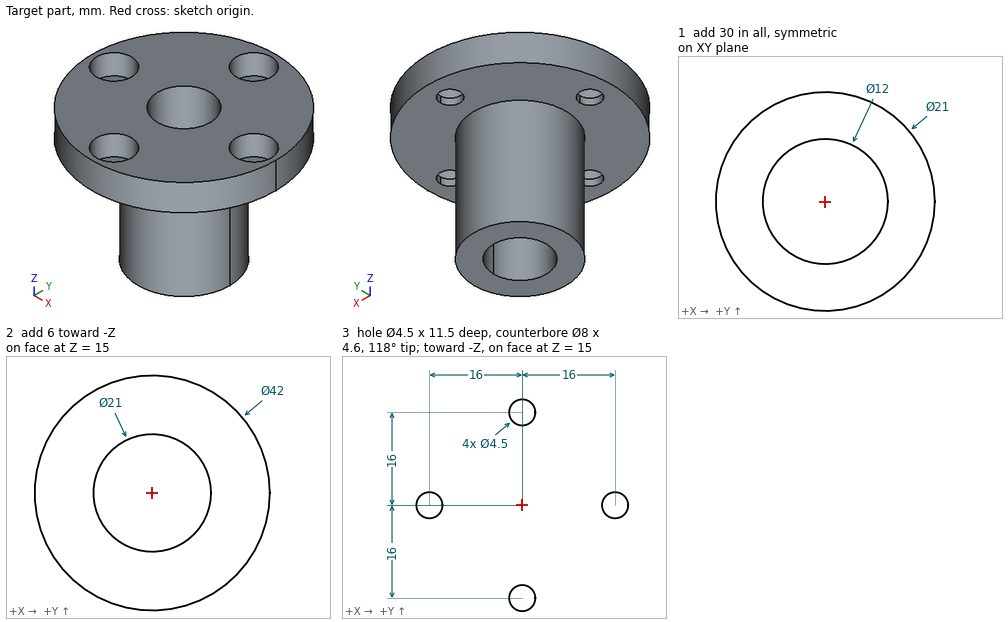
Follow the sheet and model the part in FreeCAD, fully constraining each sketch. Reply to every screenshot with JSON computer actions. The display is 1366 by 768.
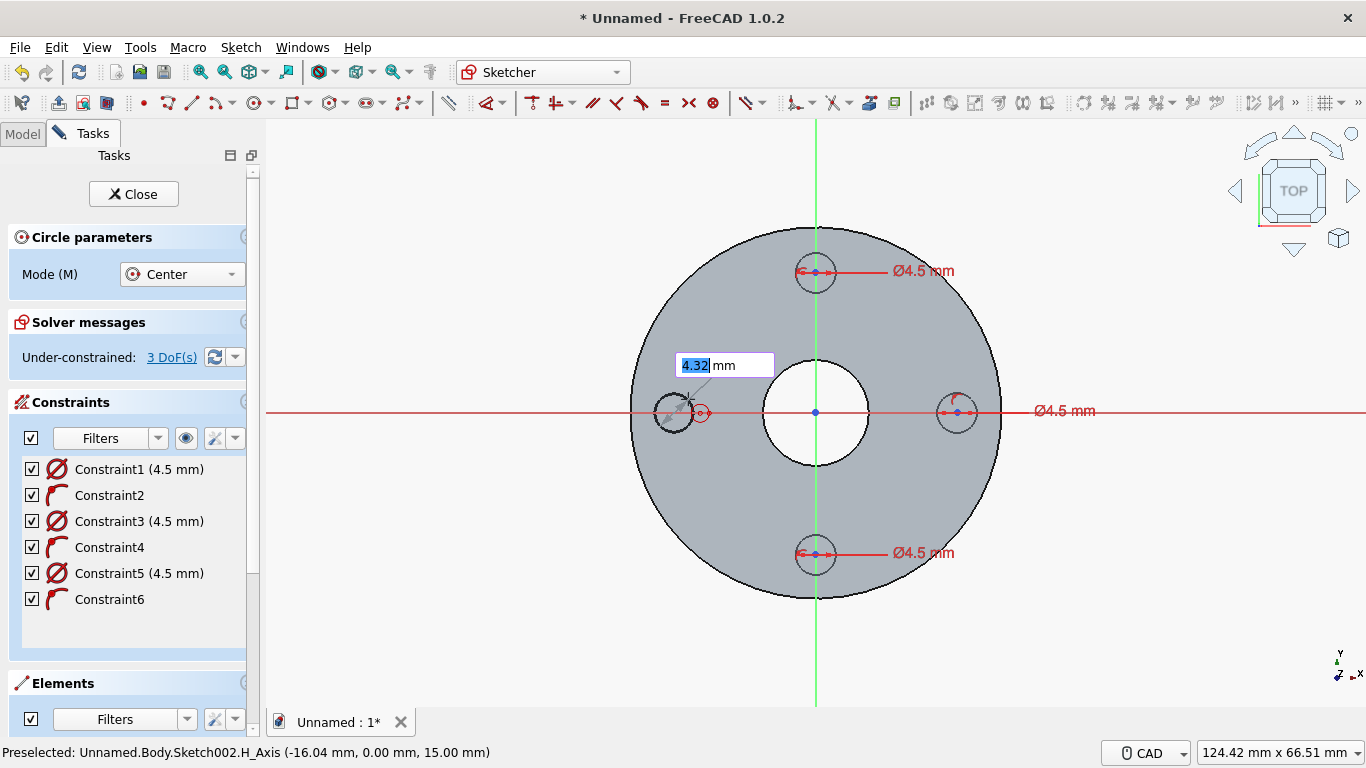
{"action": "type", "text": "4.5"}
{"action": "key", "text": "Return"}
{"action": "key", "text": "Escape"}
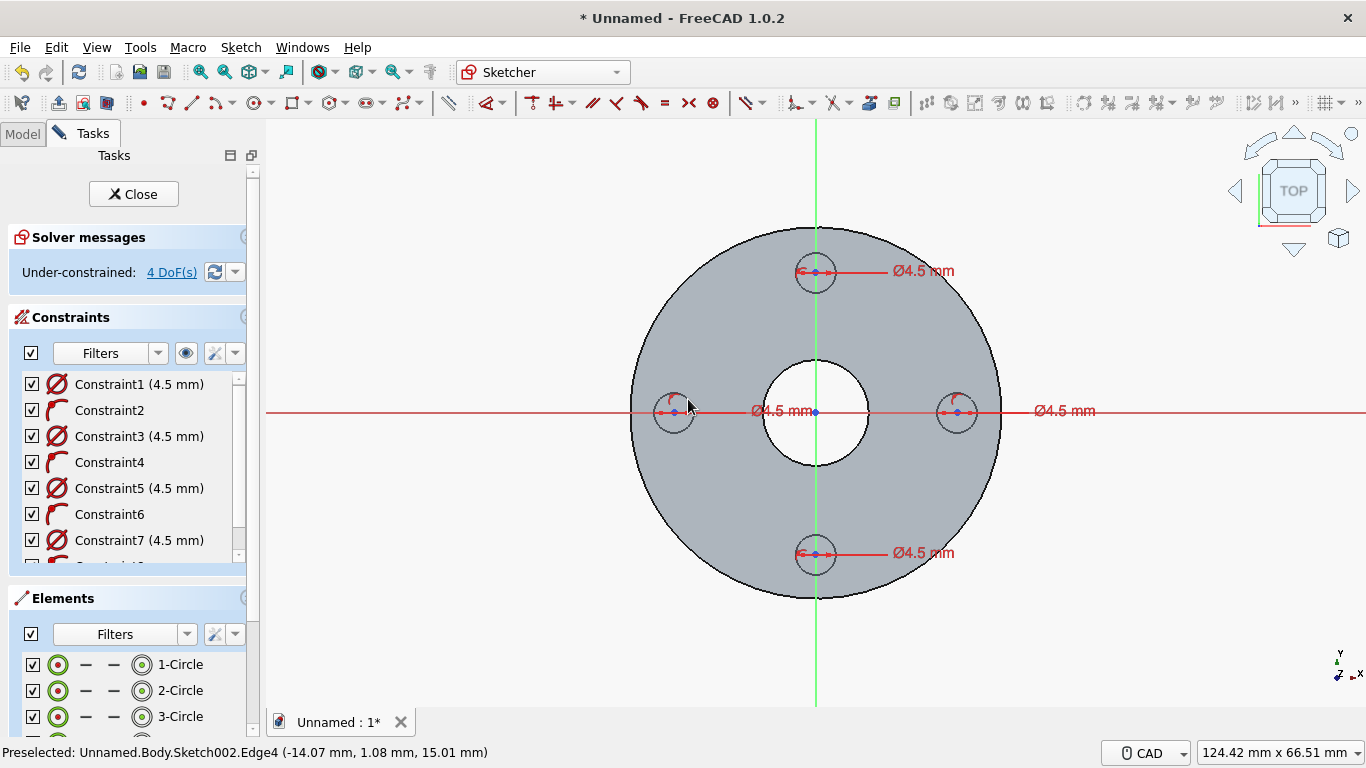
{"action": "left_click", "coordinate": [486, 104]}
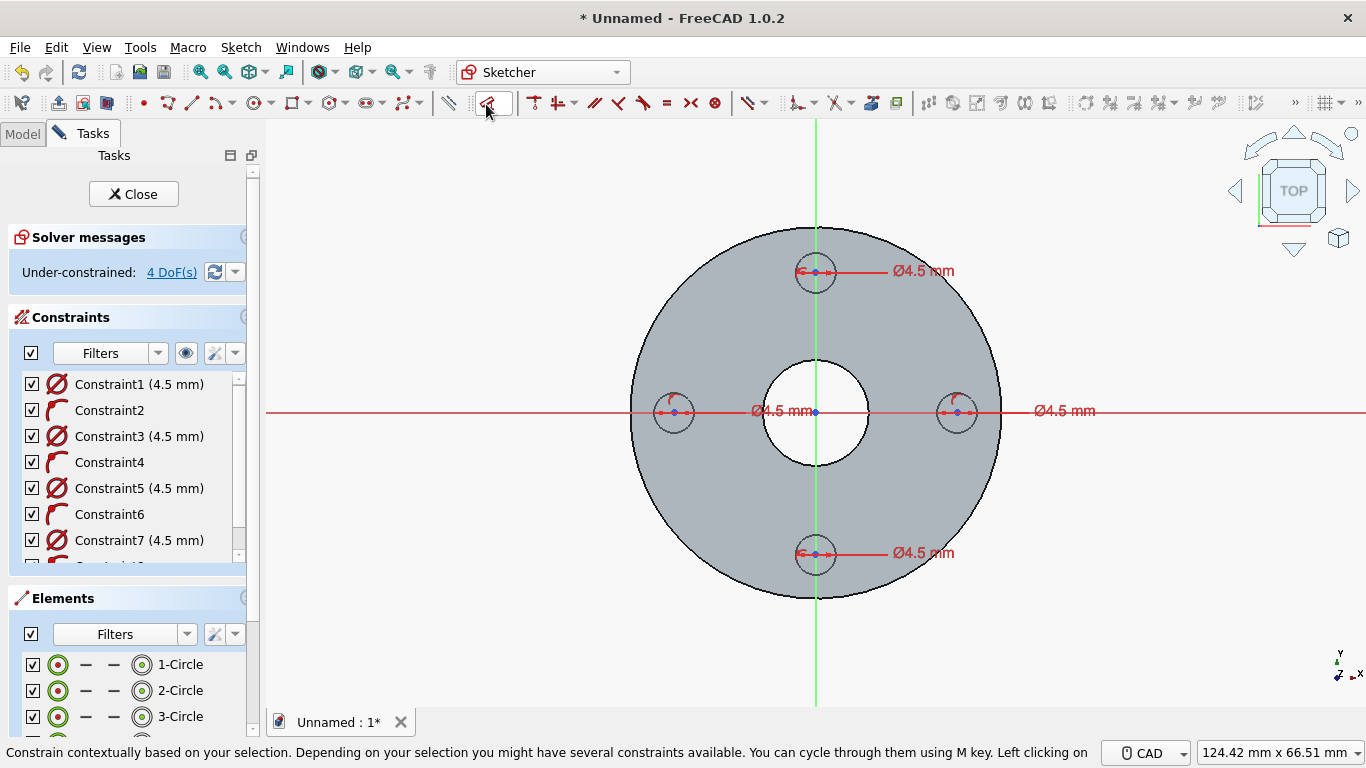
{"action": "left_click", "coordinate": [816, 273]}
{"action": "left_click", "coordinate": [850, 343]}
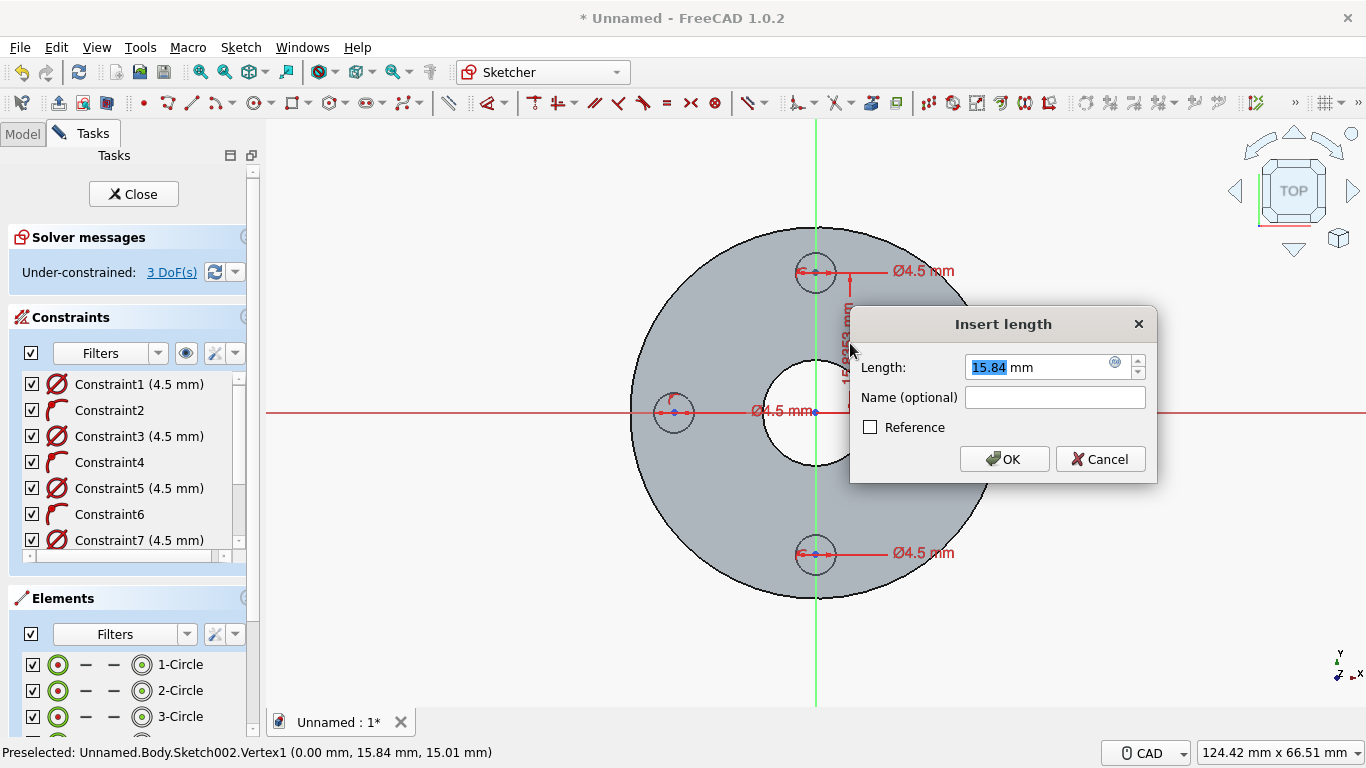
{"action": "type", "text": "16"}
{"action": "key", "text": "Return"}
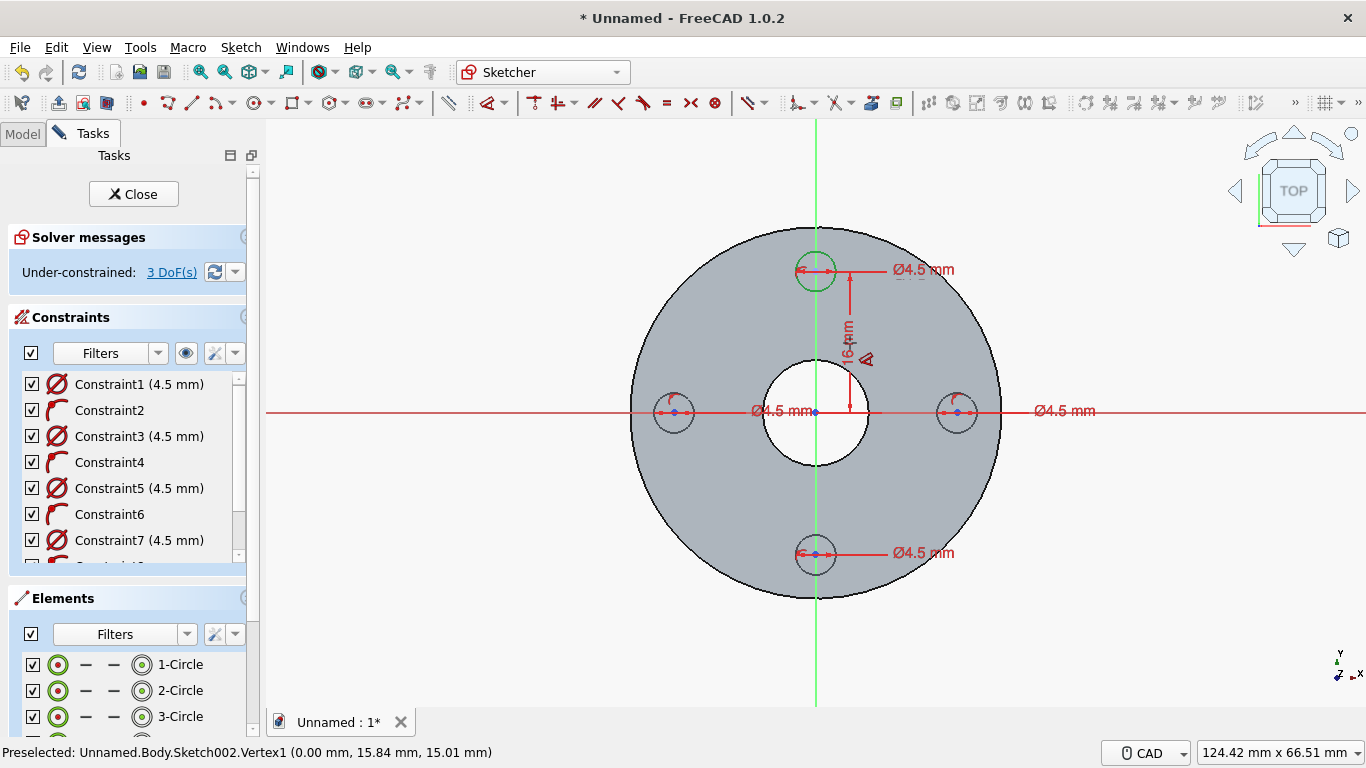
{"action": "left_click", "coordinate": [957, 413]}
{"action": "left_click", "coordinate": [886, 447]}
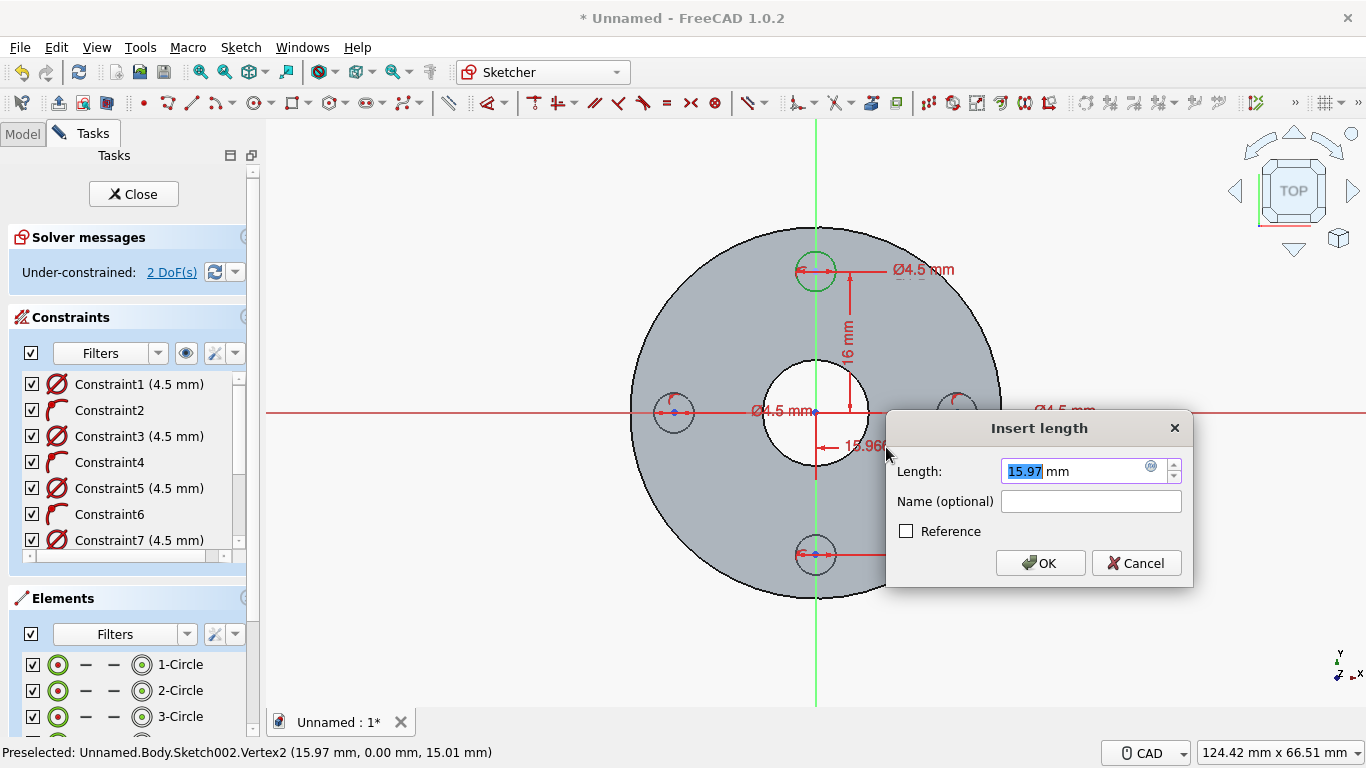
{"action": "type", "text": "16"}
{"action": "key", "text": "Return"}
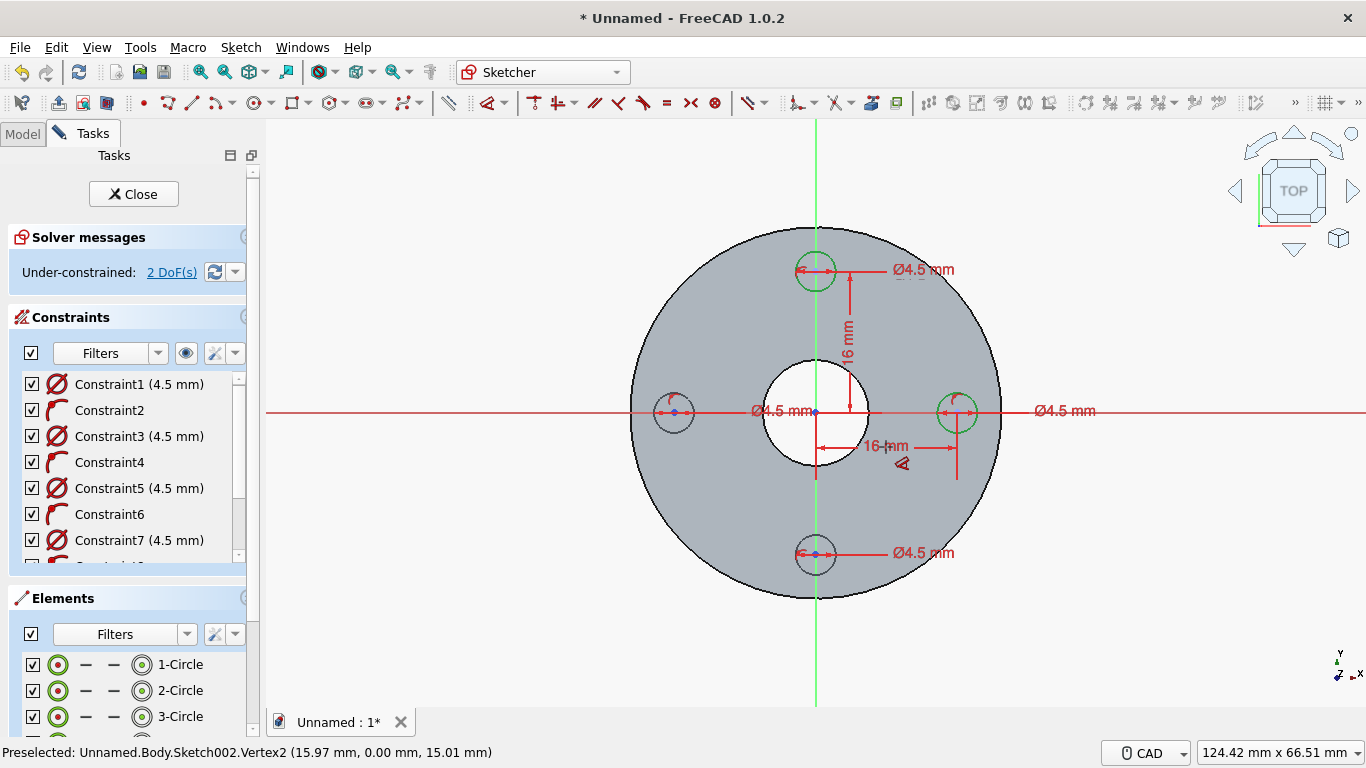
{"action": "left_click", "coordinate": [816, 555]}
{"action": "left_click", "coordinate": [850, 484]}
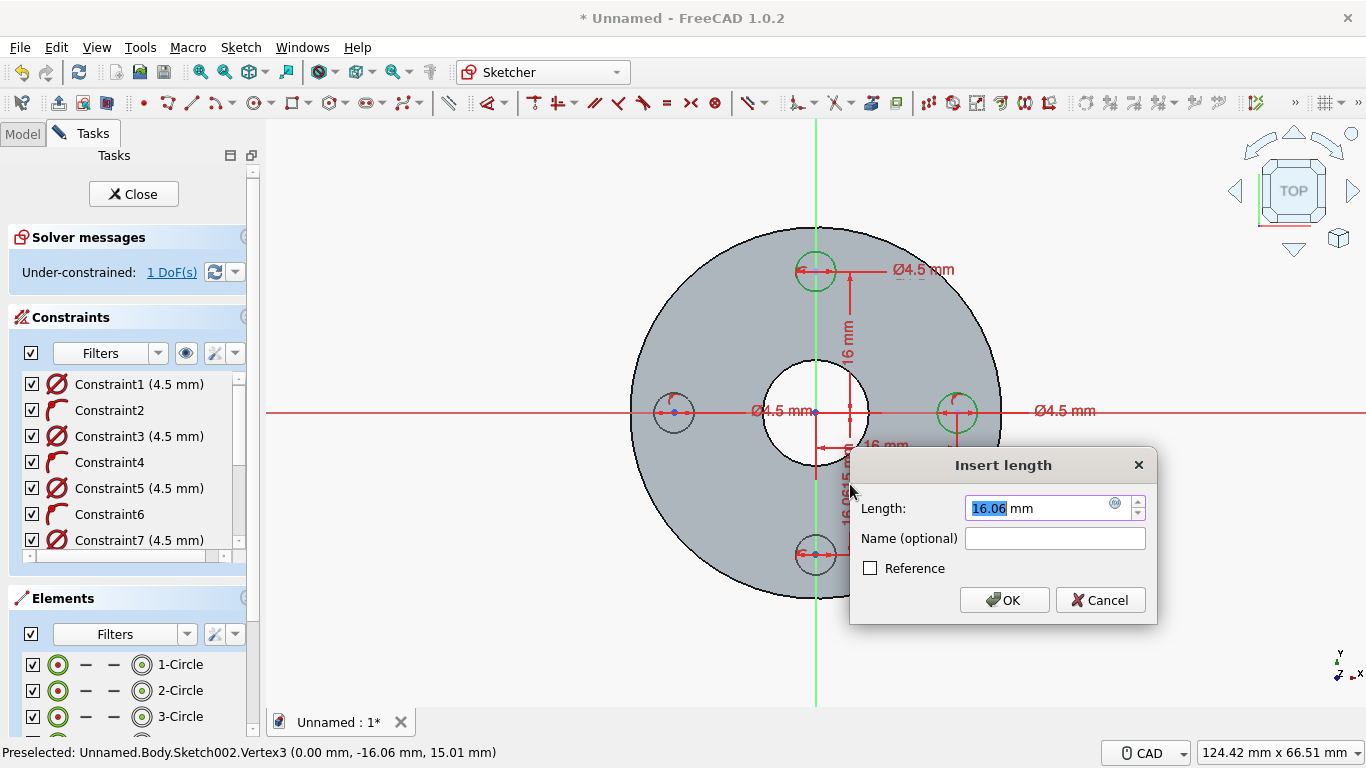
{"action": "type", "text": "16"}
{"action": "key", "text": "Return"}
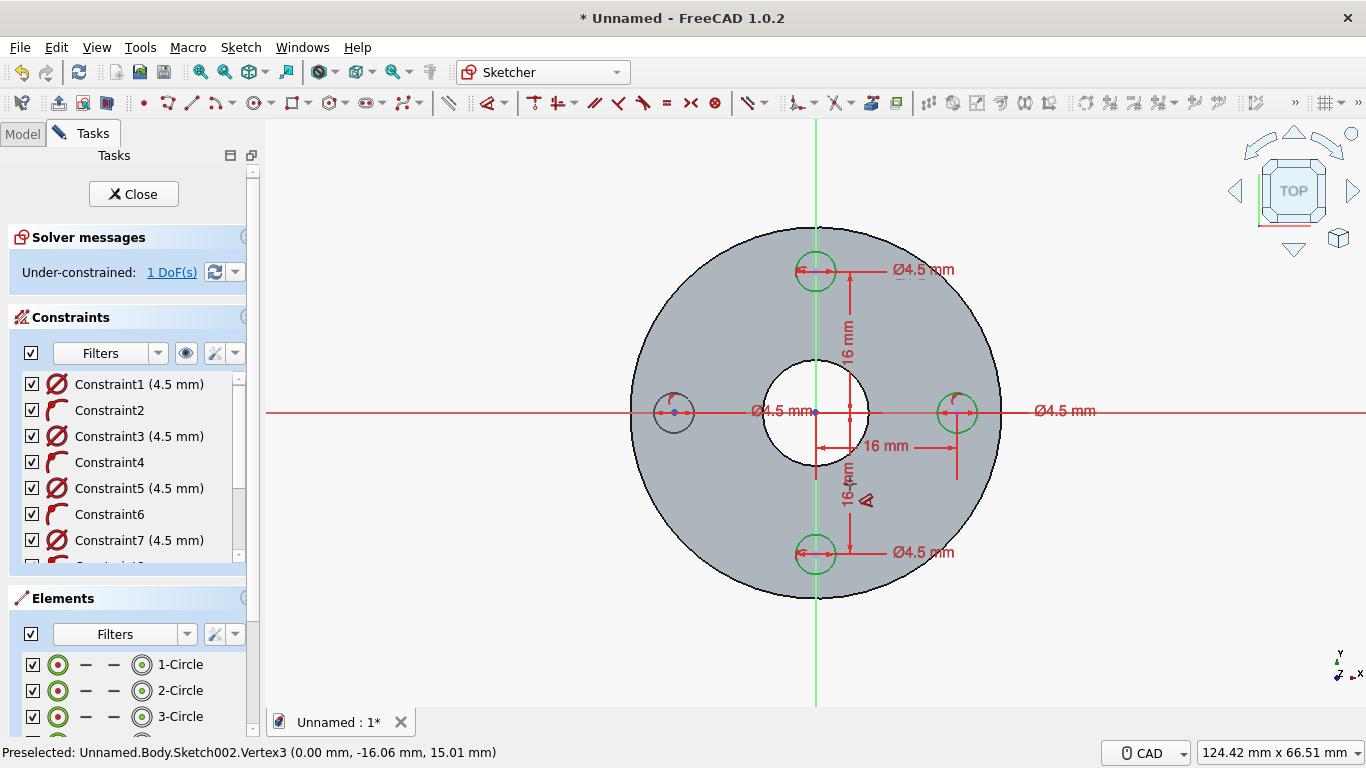
{"action": "left_click", "coordinate": [674, 413]}
{"action": "left_click", "coordinate": [745, 447]}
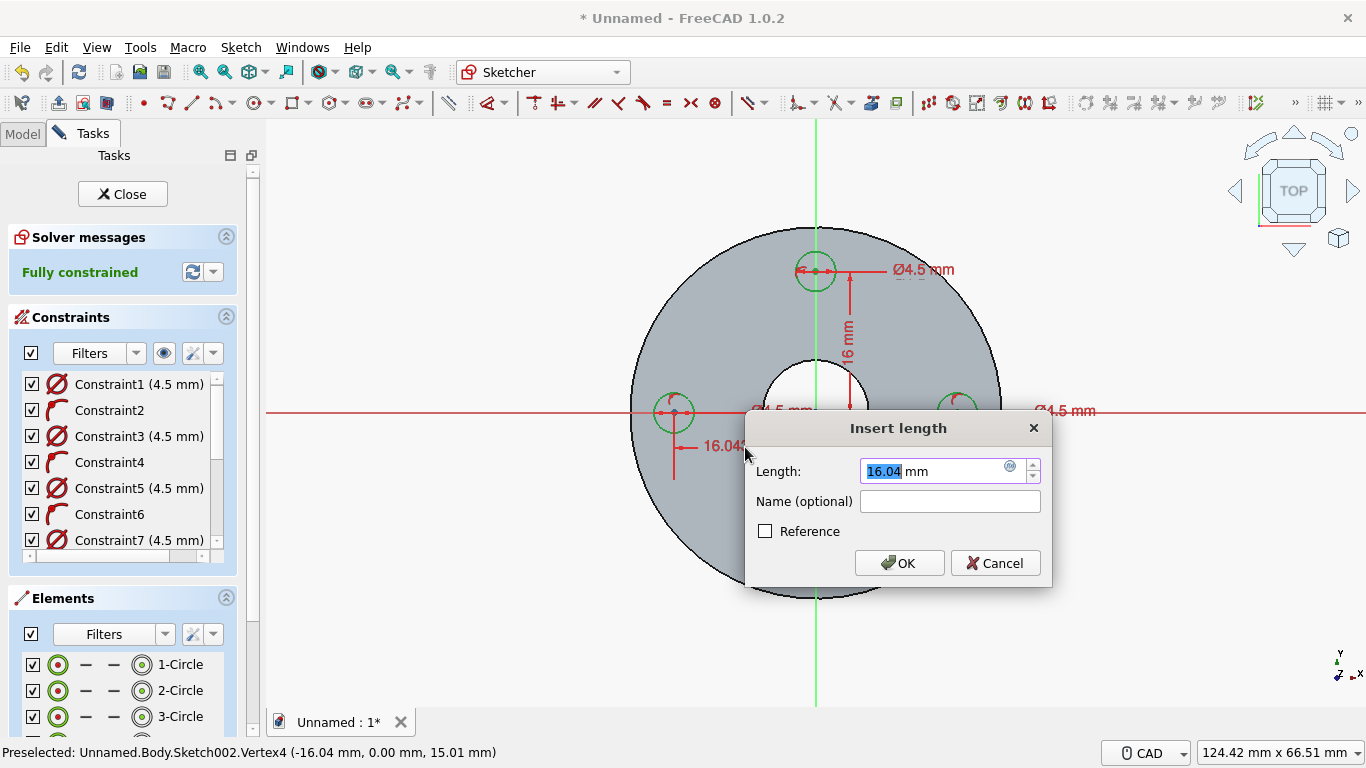
{"action": "type", "text": "16"}
{"action": "key", "text": "Return"}
{"action": "key", "text": "Escape"}